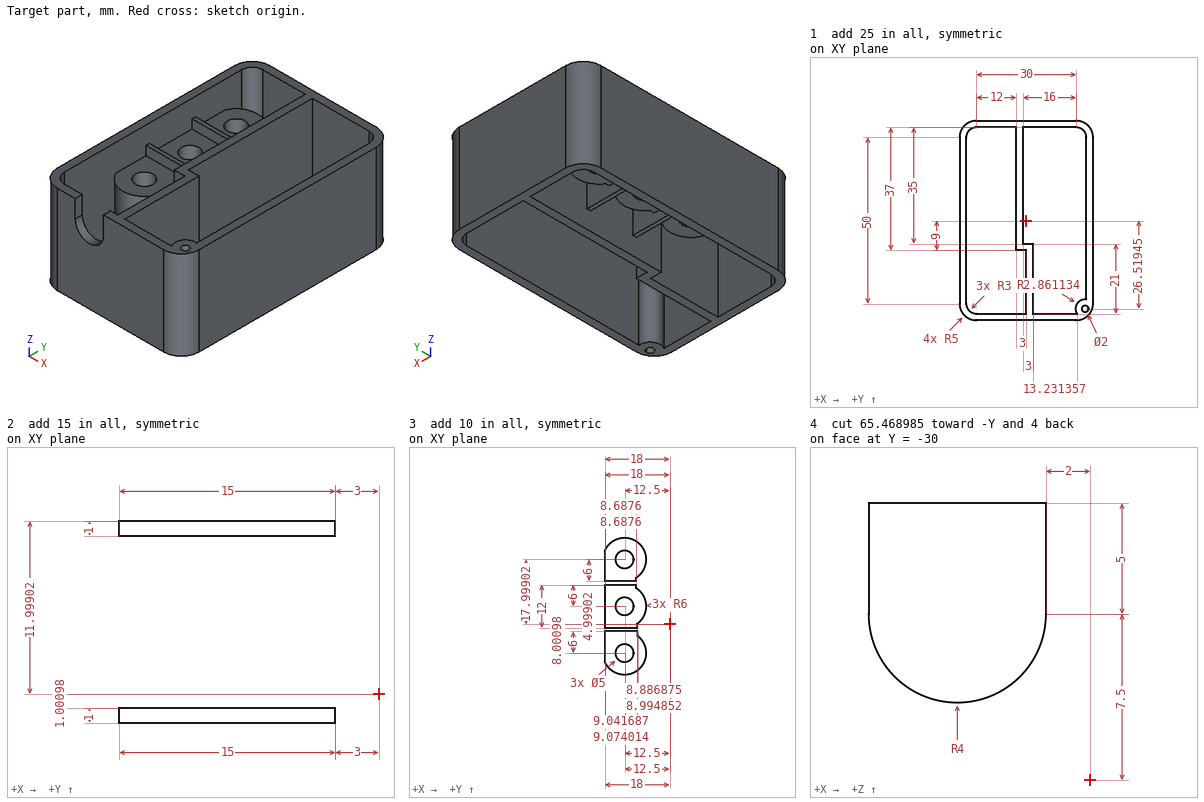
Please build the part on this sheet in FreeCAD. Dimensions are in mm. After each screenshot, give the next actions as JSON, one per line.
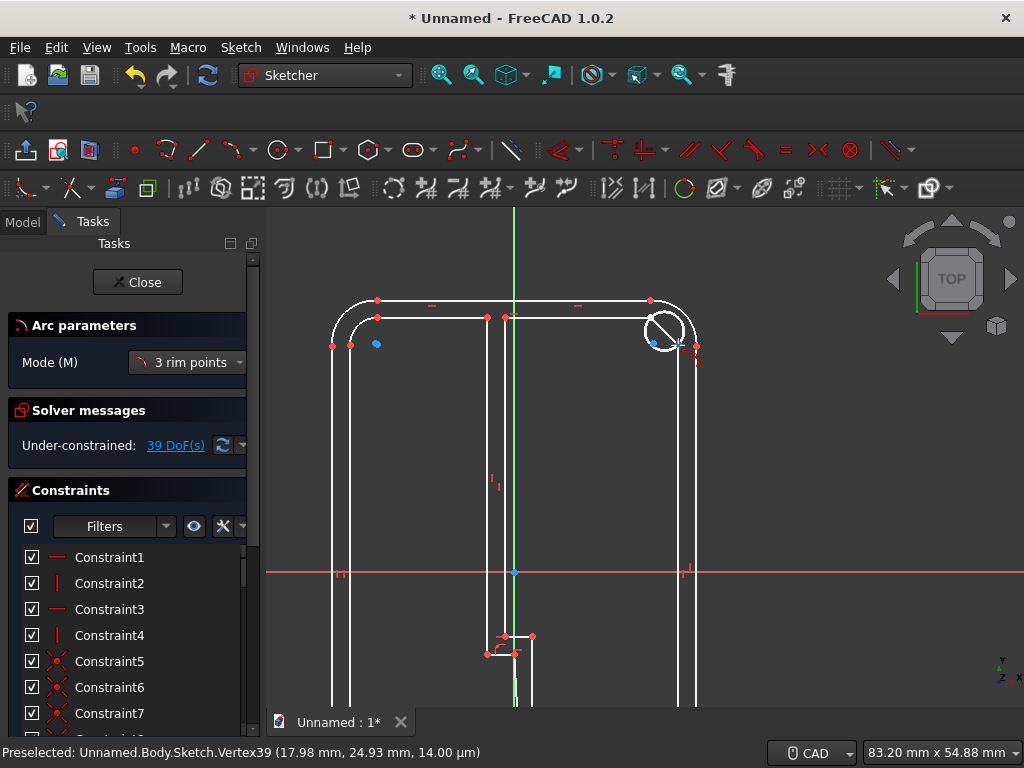
{"action": "scroll", "coordinate": [670, 325], "scroll_direction": "up", "scroll_amount": 4}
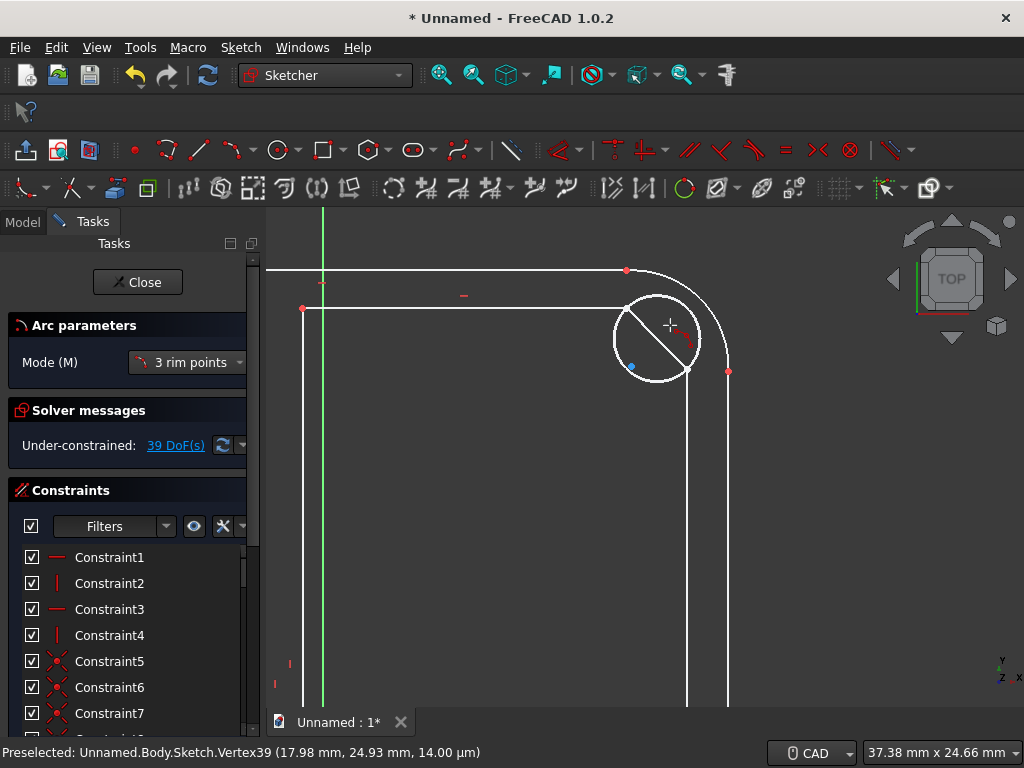
{"action": "left_click", "coordinate": [670, 325]}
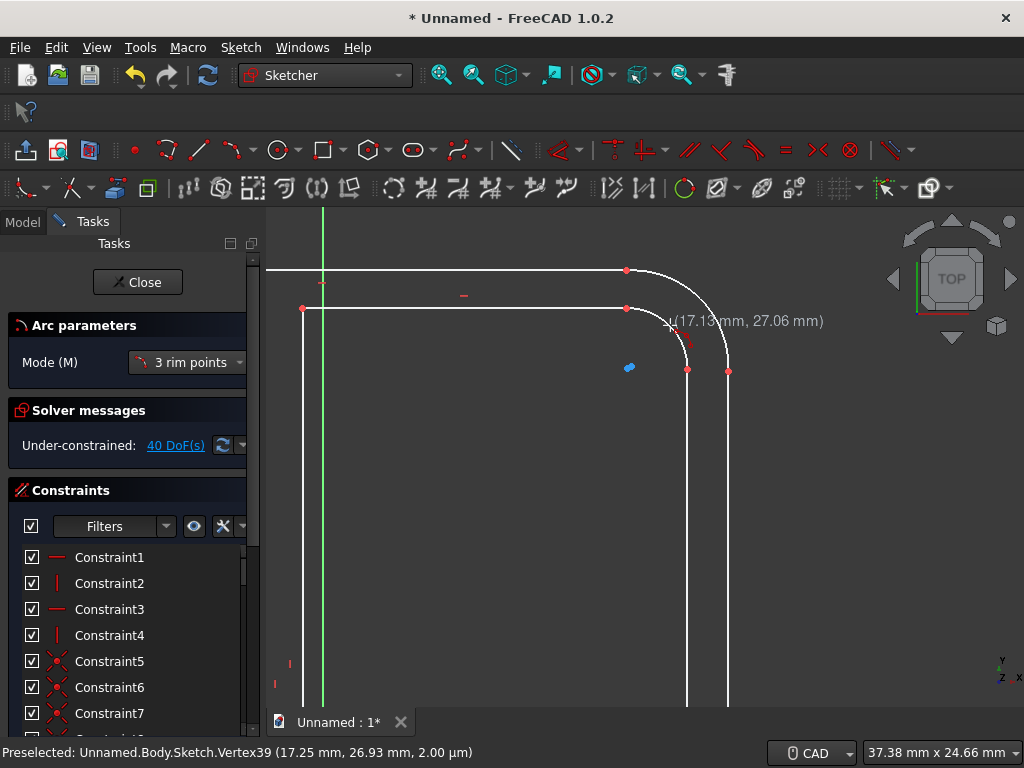
{"action": "left_click", "coordinate": [278, 150]}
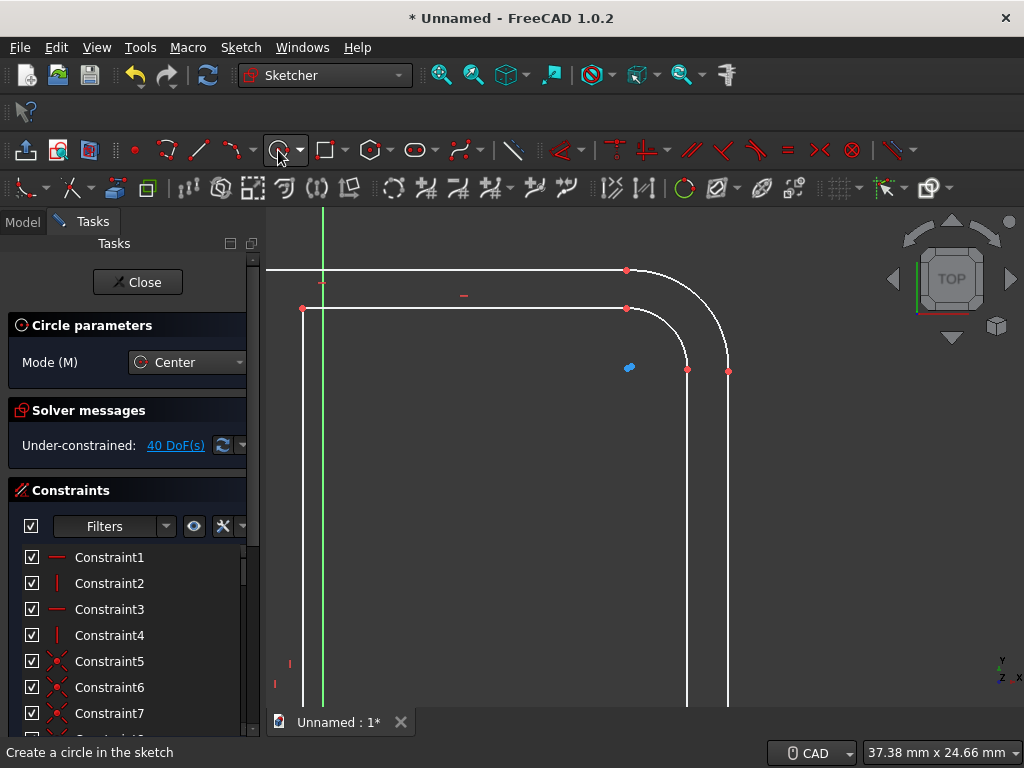
{"action": "scroll", "coordinate": [660, 320], "scroll_direction": "down", "scroll_amount": 7}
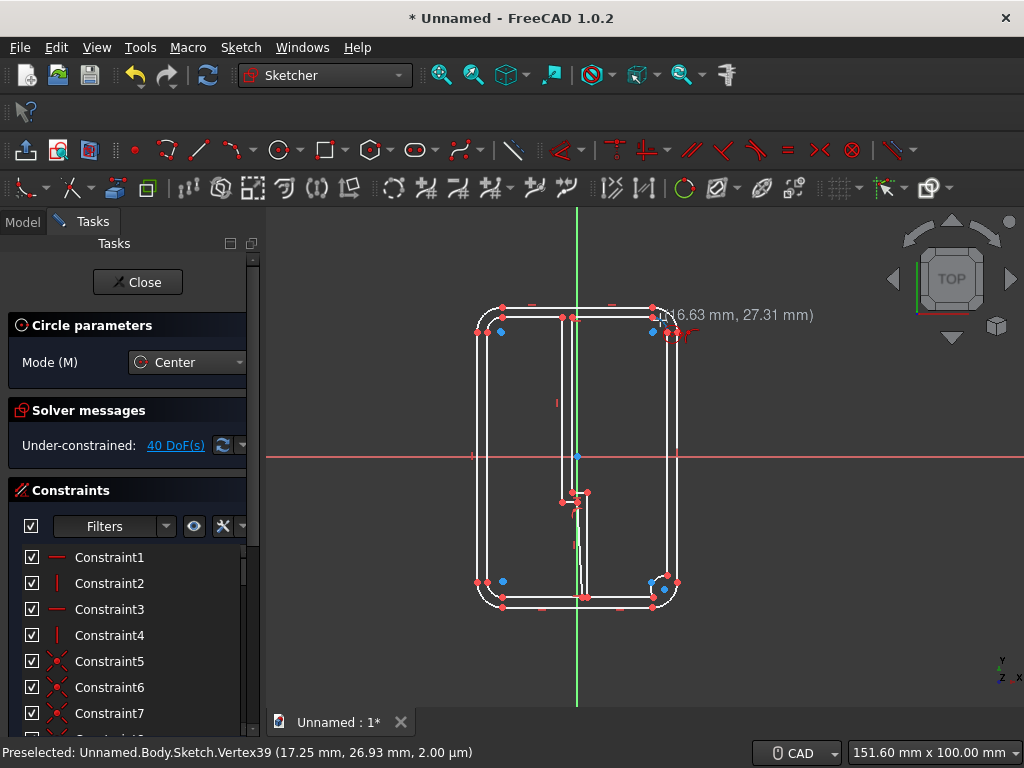
{"action": "scroll", "coordinate": [666, 590], "scroll_direction": "up", "scroll_amount": 8}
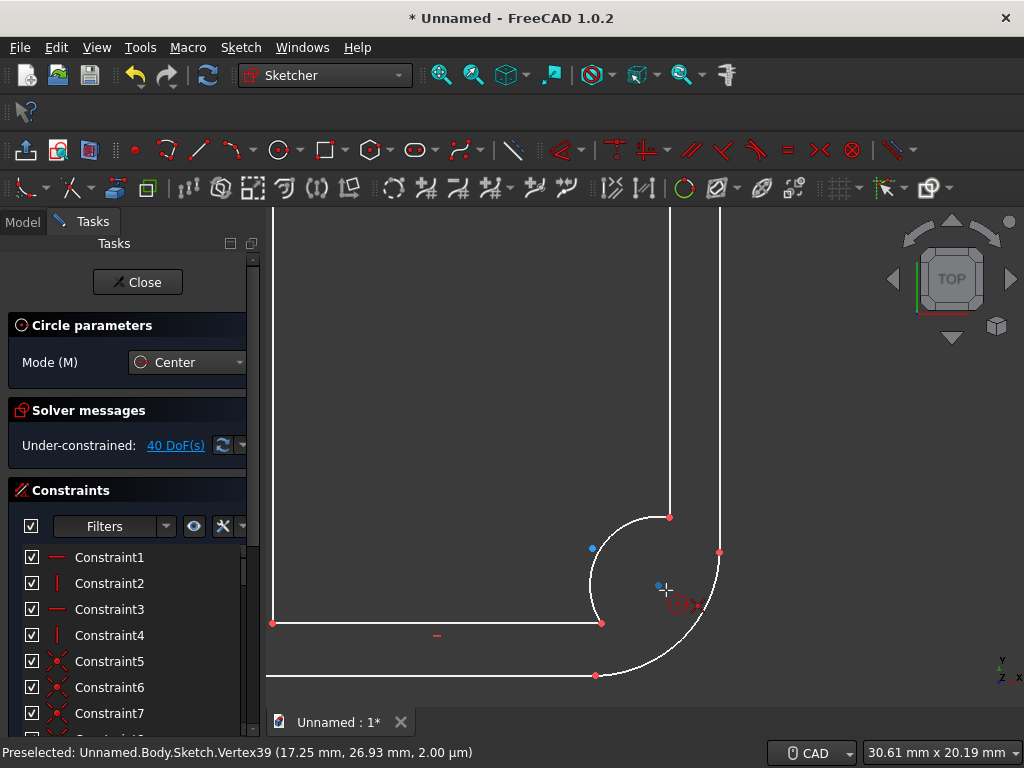
{"action": "scroll", "coordinate": [666, 591], "scroll_direction": "down", "scroll_amount": 8}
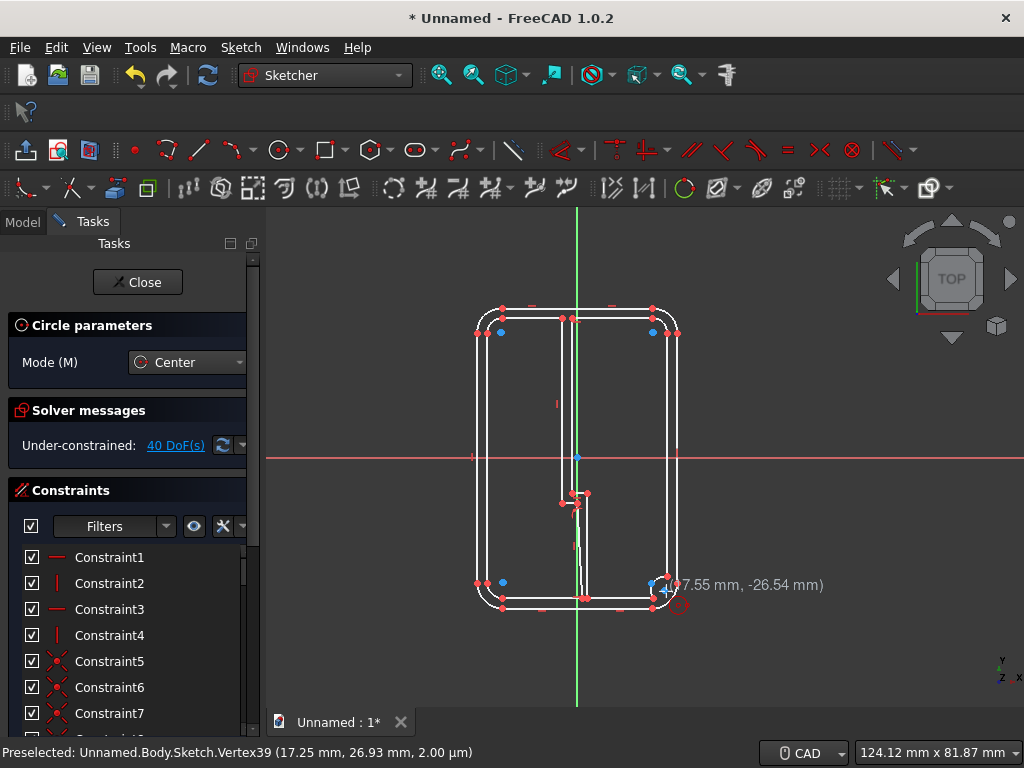
{"action": "scroll", "coordinate": [666, 590], "scroll_direction": "up", "scroll_amount": 3}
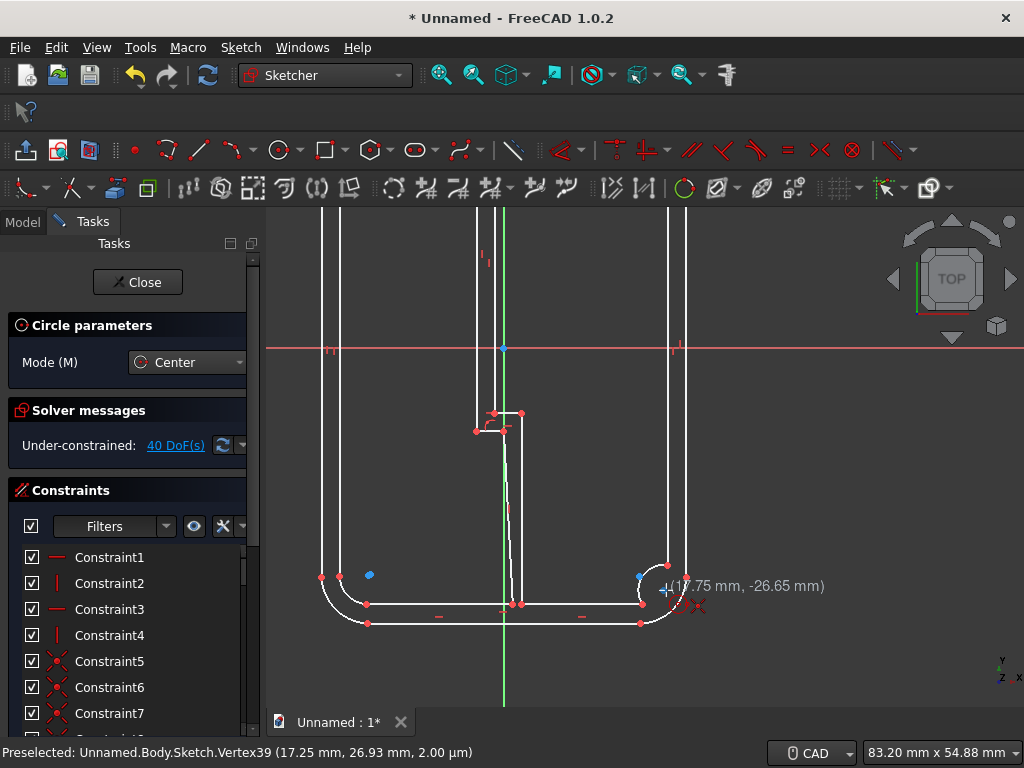
{"action": "left_click", "coordinate": [665, 590]}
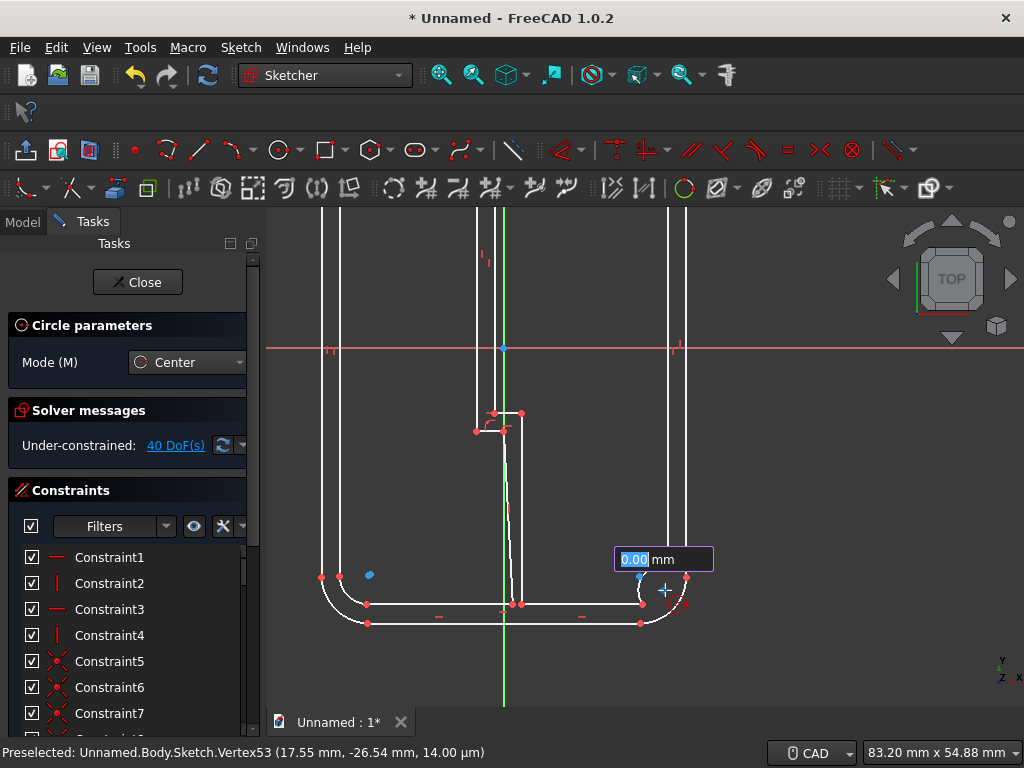
{"action": "scroll", "coordinate": [673, 587], "scroll_direction": "up", "scroll_amount": 3}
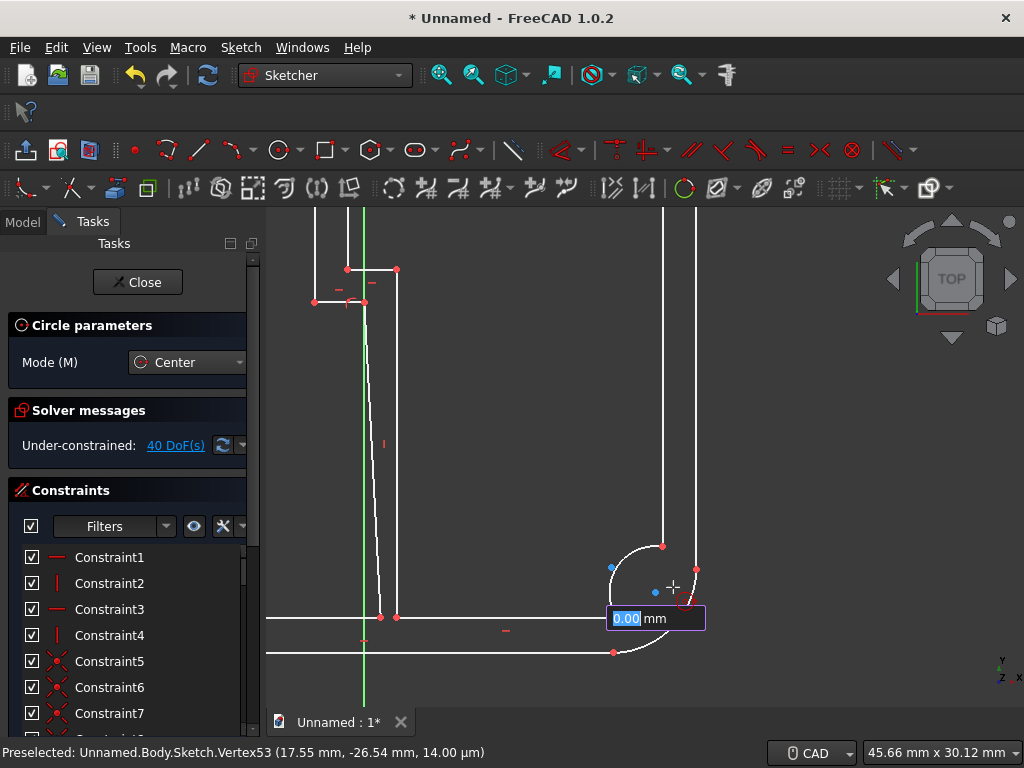
{"action": "left_click", "coordinate": [673, 586]}
{"action": "key", "text": "Escape"}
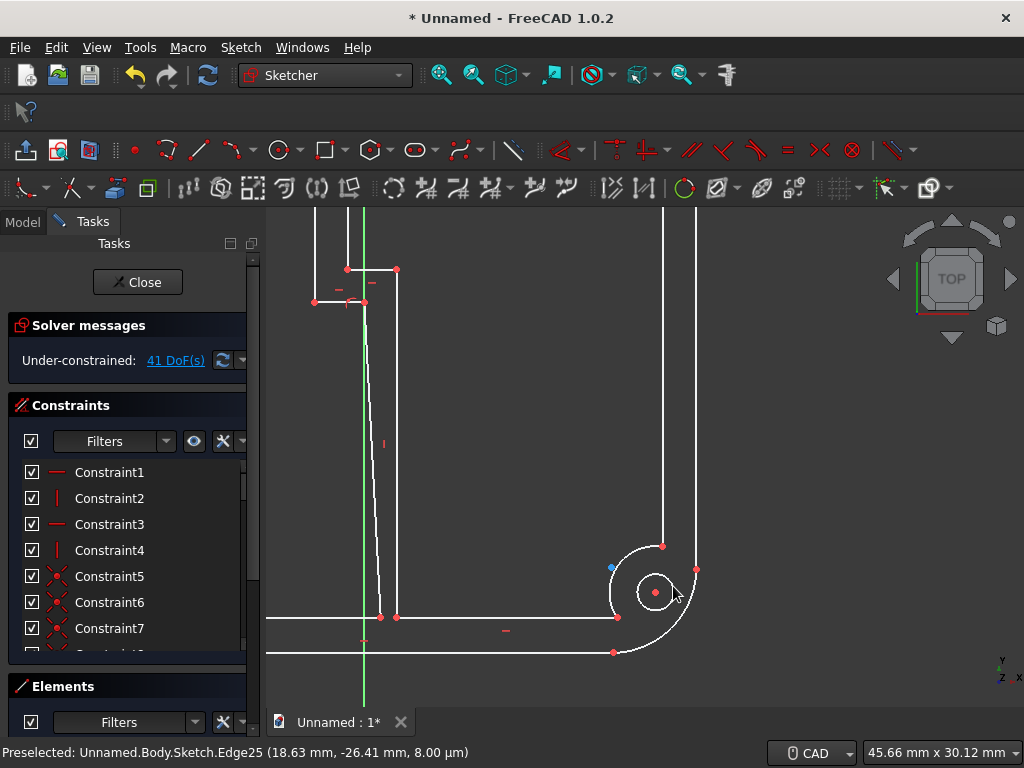
{"action": "scroll", "coordinate": [668, 589], "scroll_direction": "down", "scroll_amount": 6}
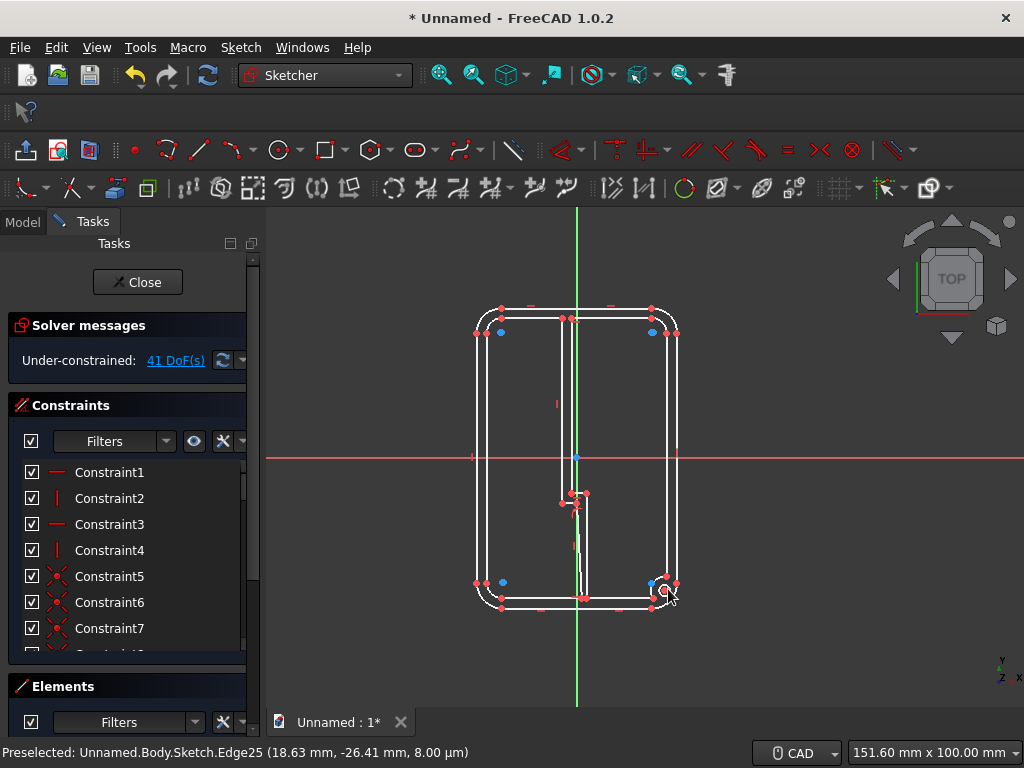
{"action": "scroll", "coordinate": [607, 309], "scroll_direction": "up", "scroll_amount": 2}